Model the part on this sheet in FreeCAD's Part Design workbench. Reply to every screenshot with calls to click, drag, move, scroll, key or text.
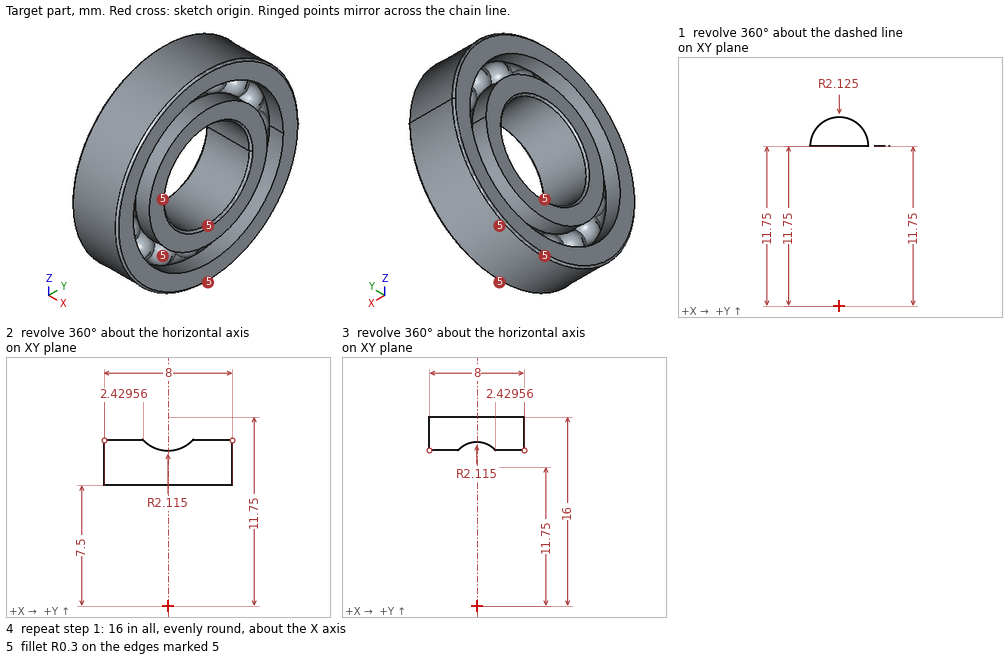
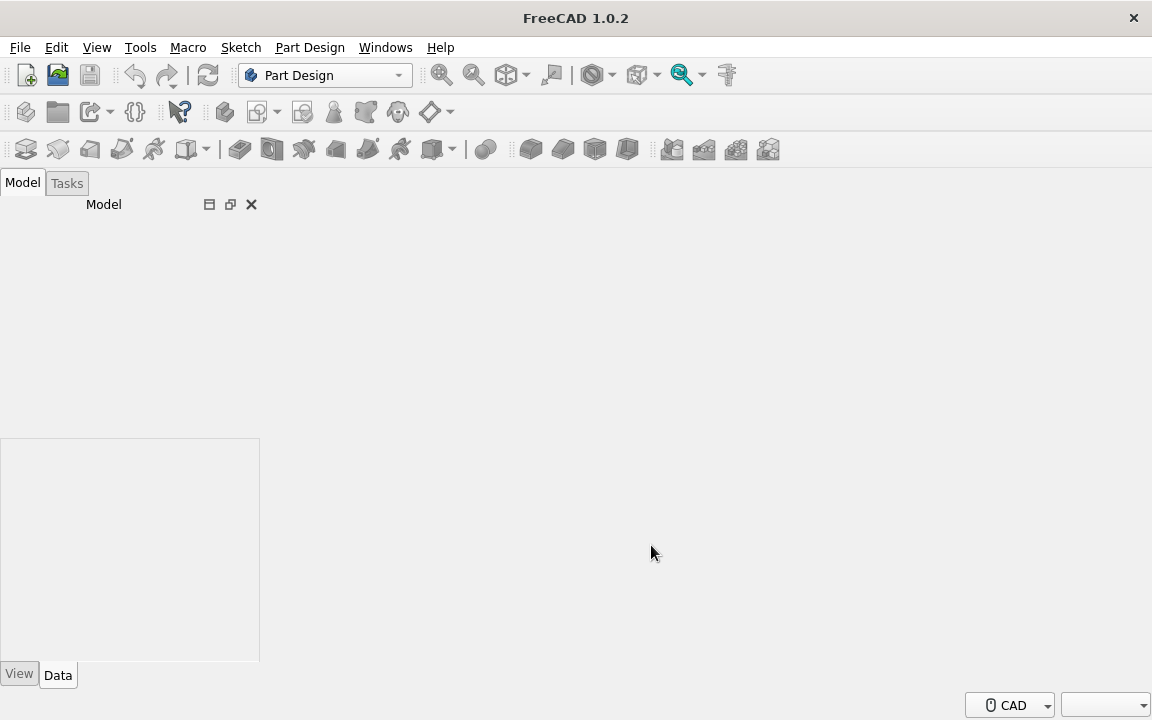
click(26, 76)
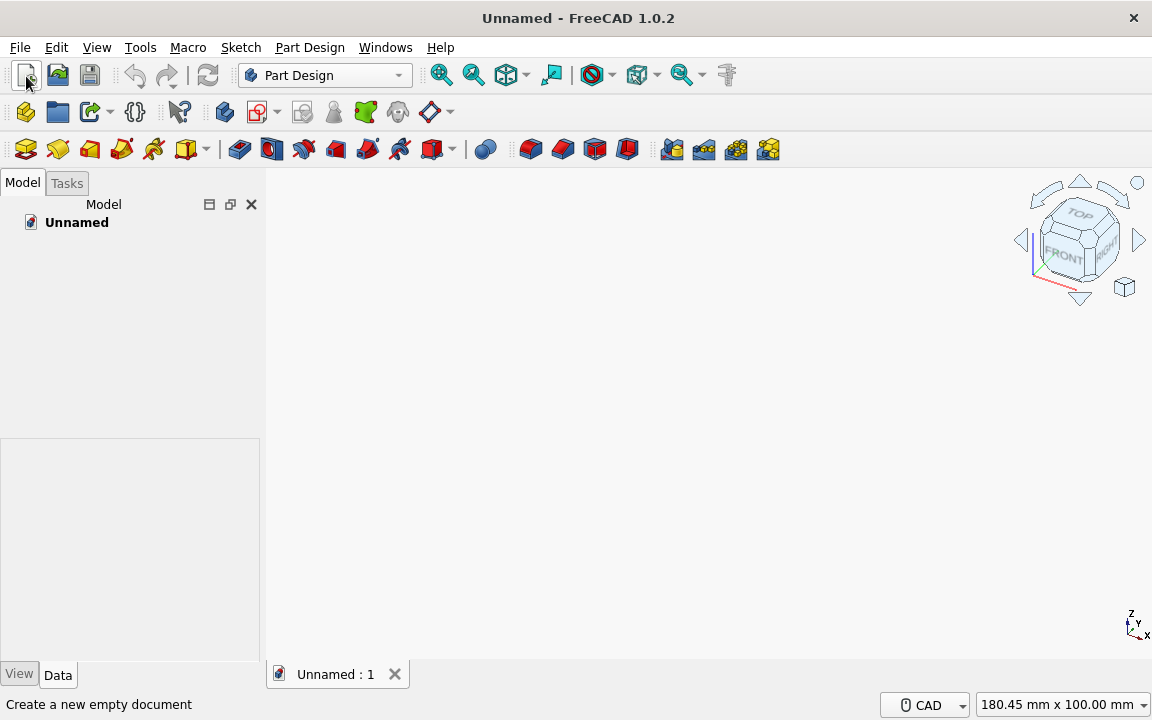
click(258, 112)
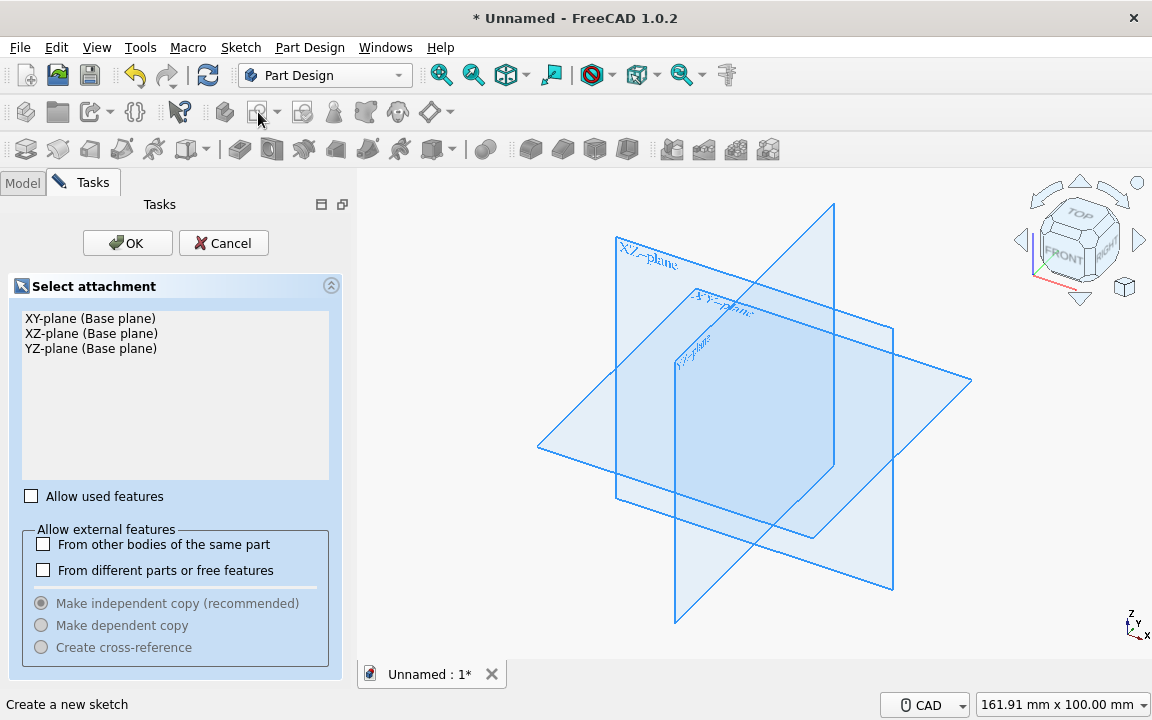
click(82, 318)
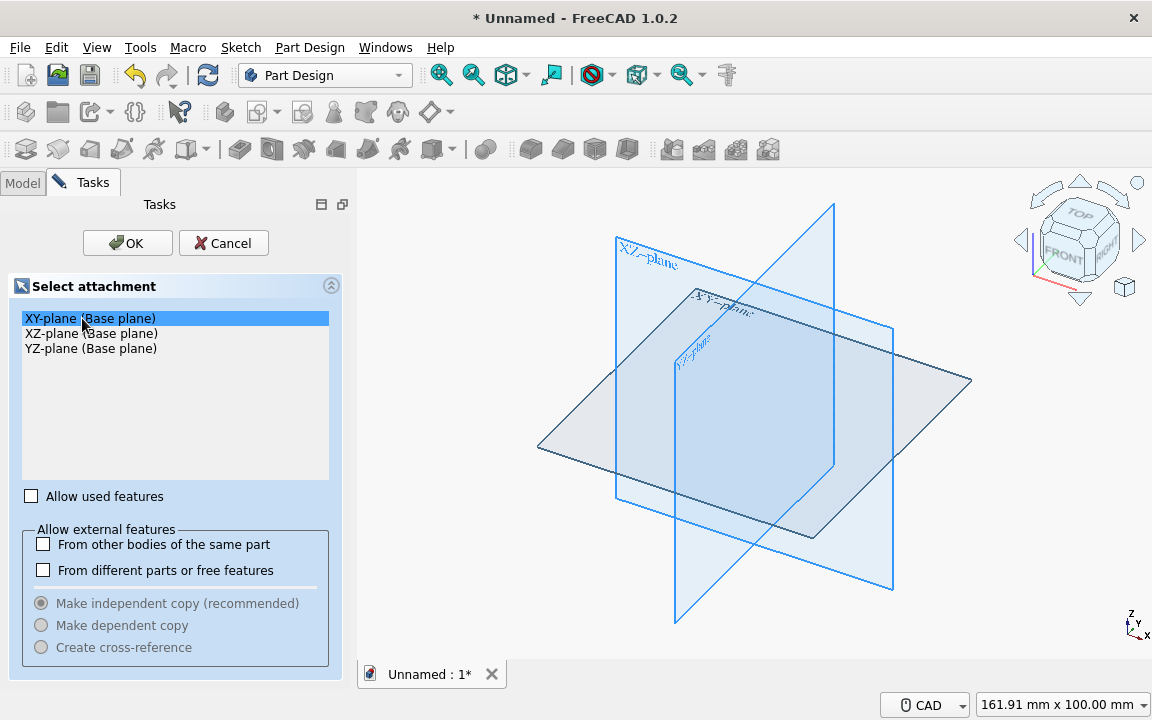
click(128, 243)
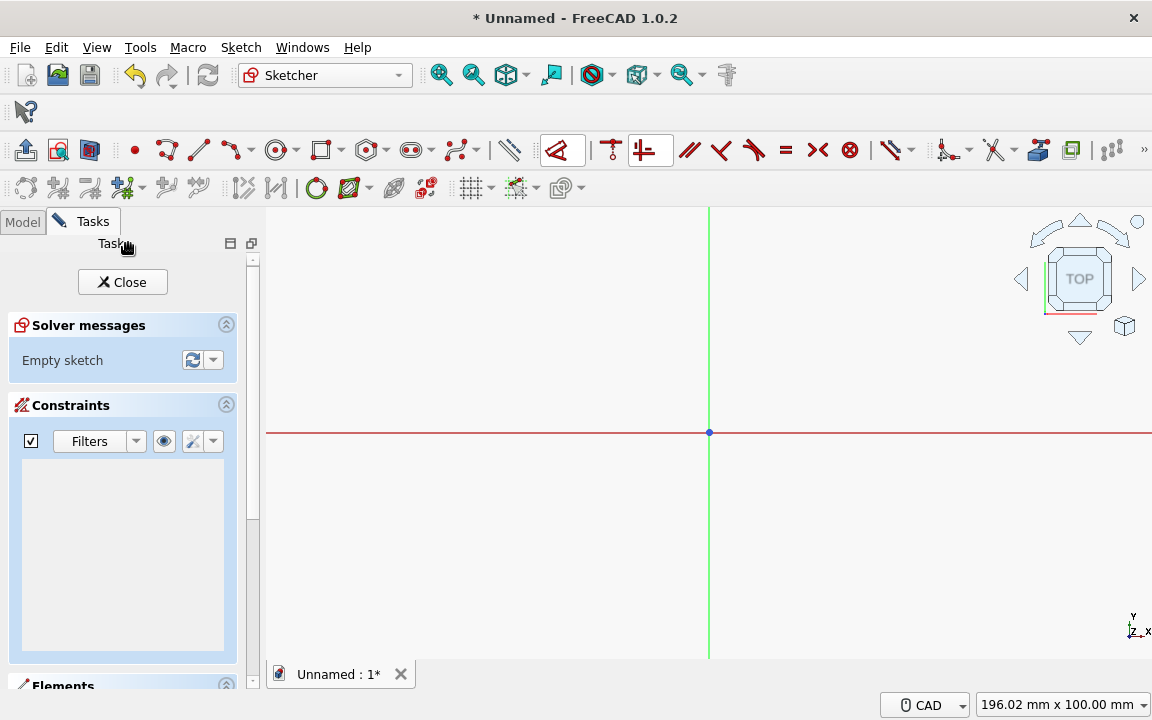
scroll(737, 391, up, 7)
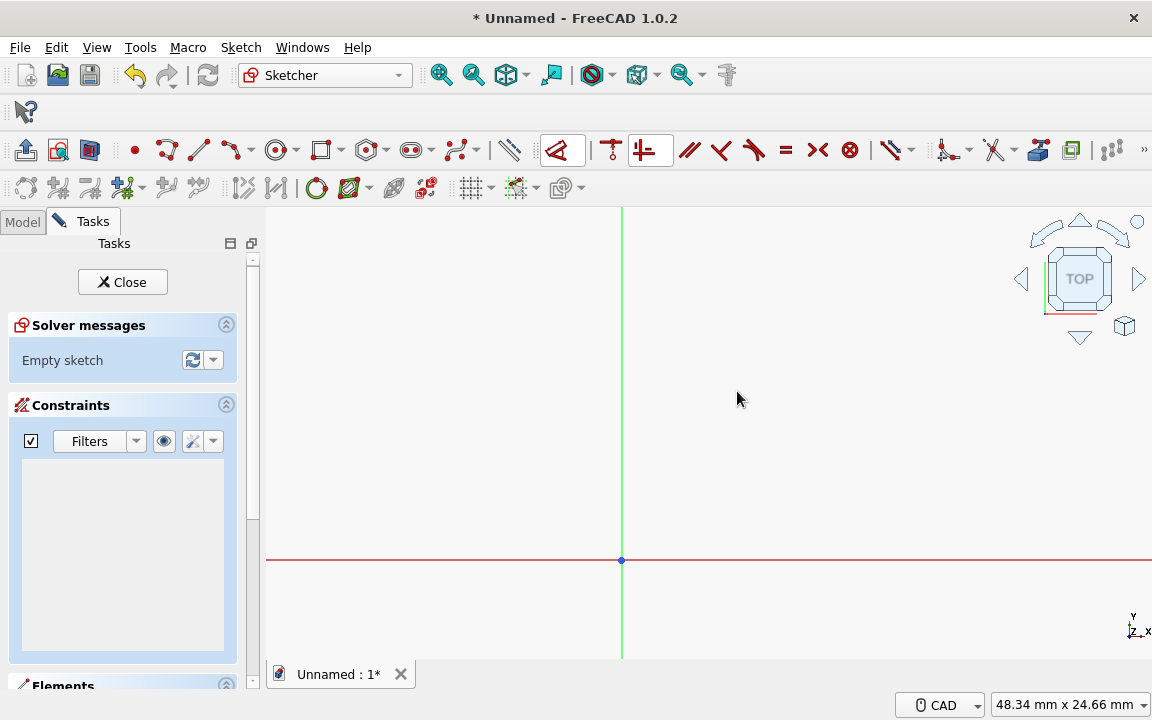
click(200, 150)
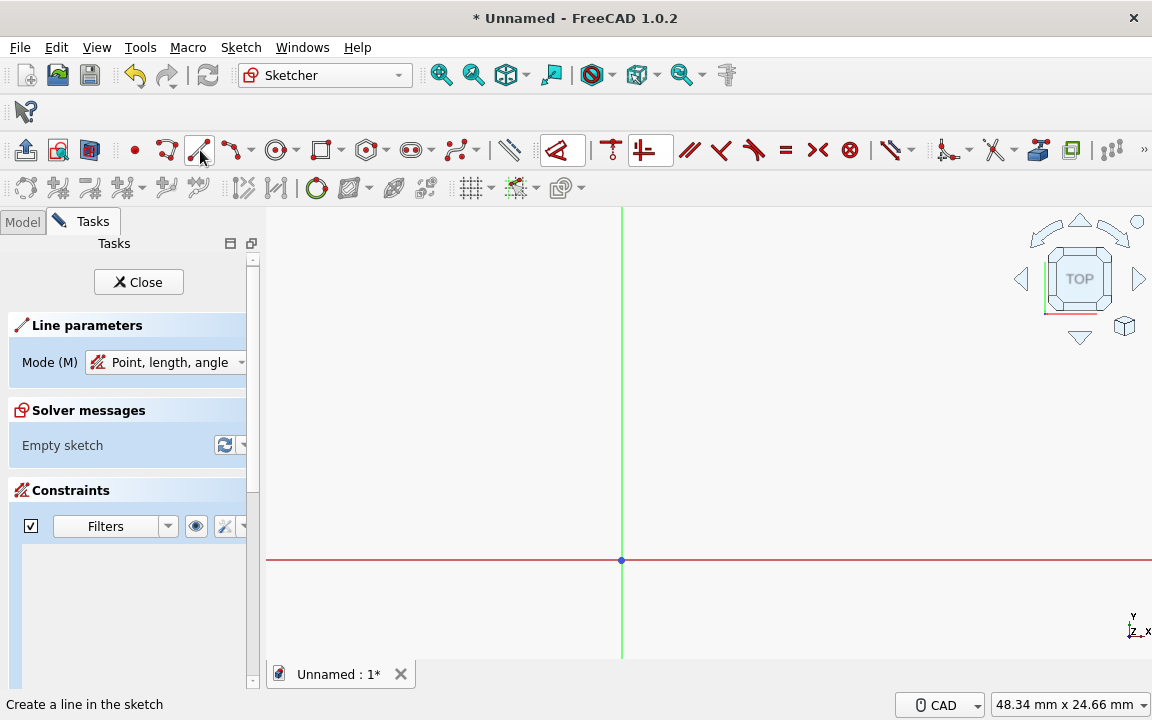
click(583, 345)
click(661, 345)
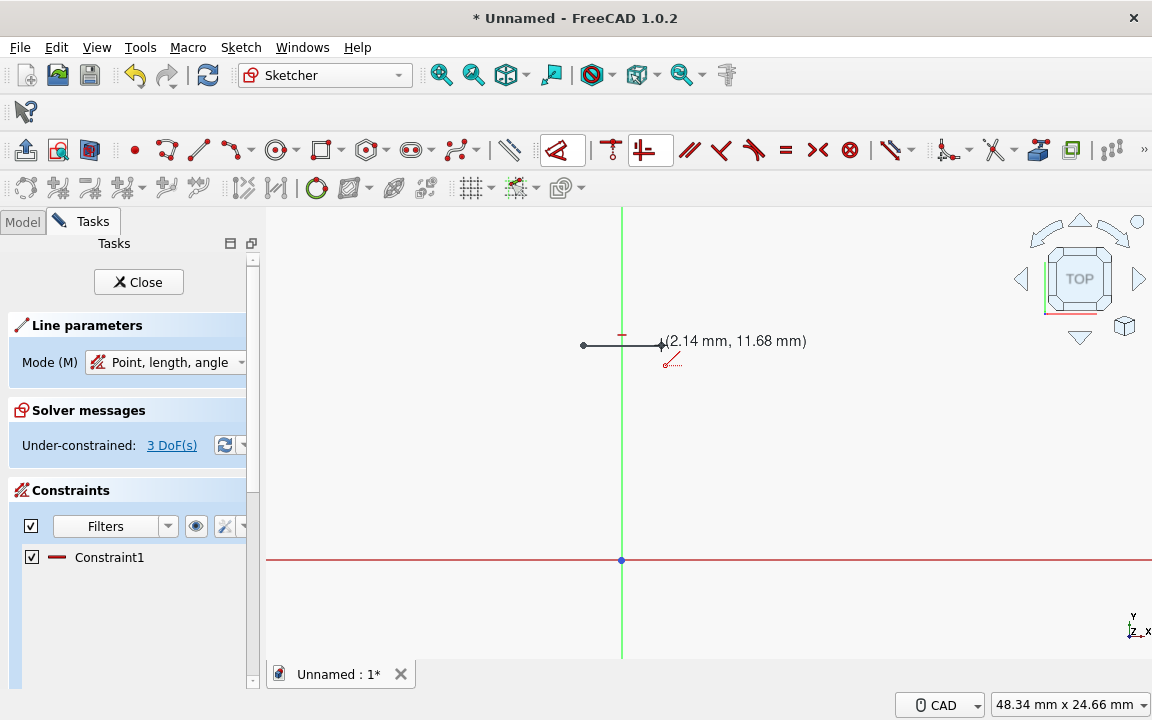
click(232, 150)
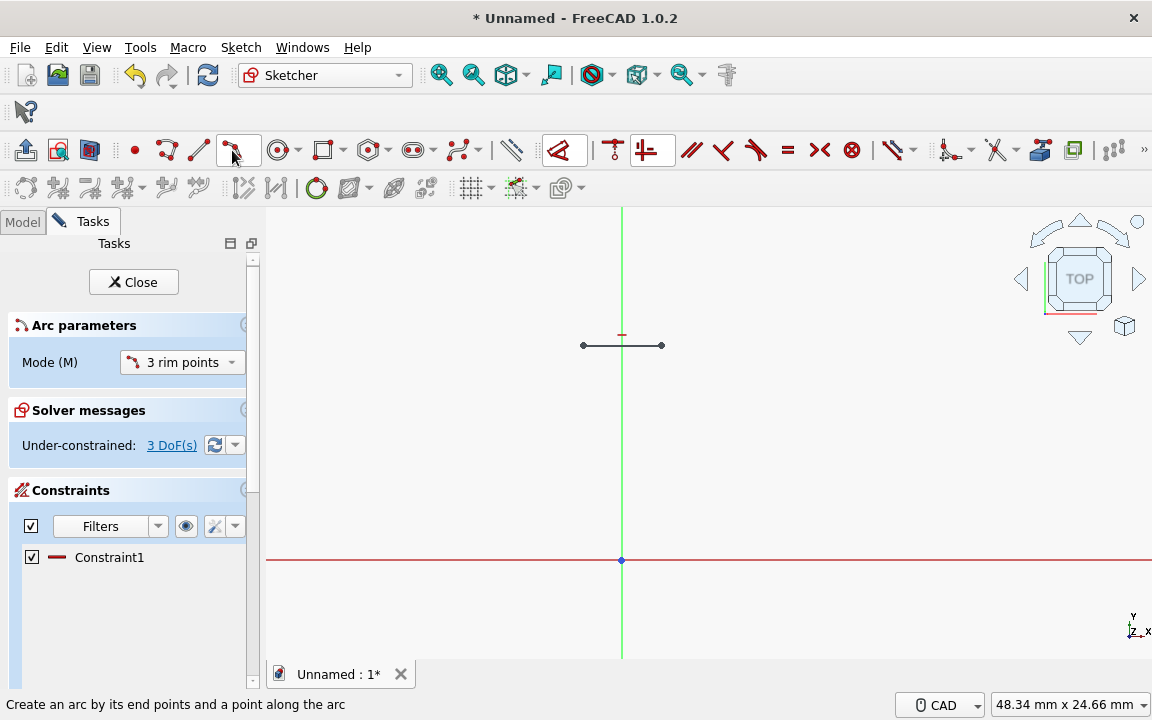
click(661, 346)
click(583, 346)
click(645, 313)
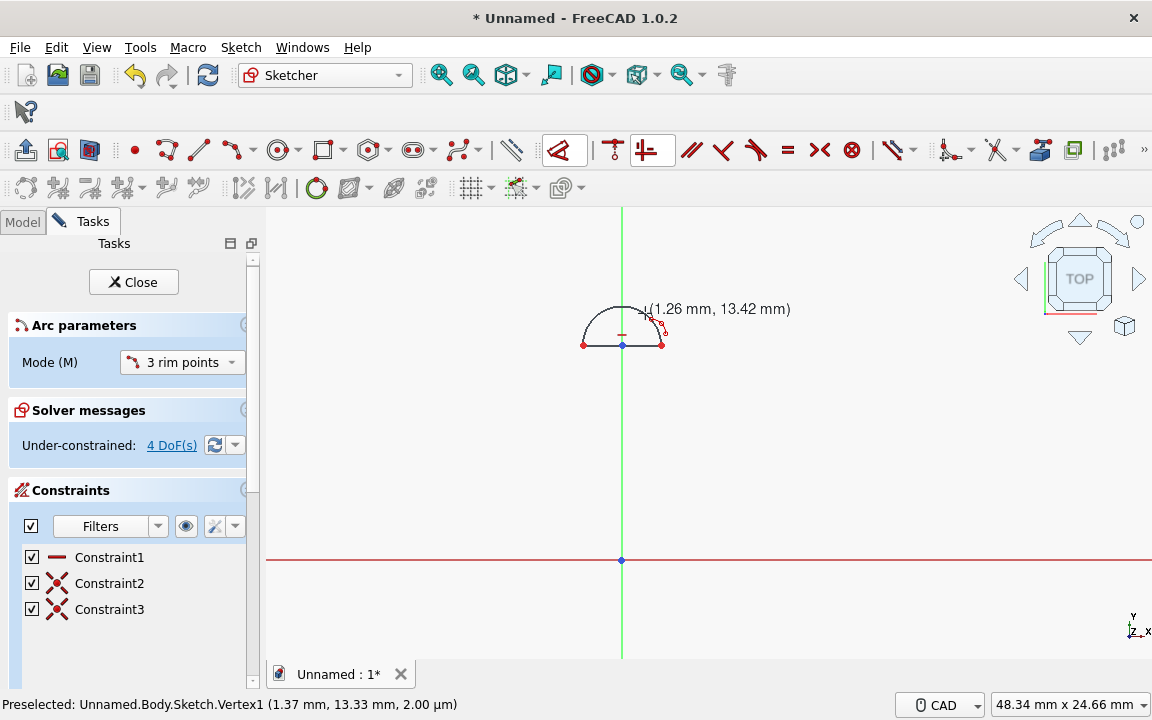
click(200, 150)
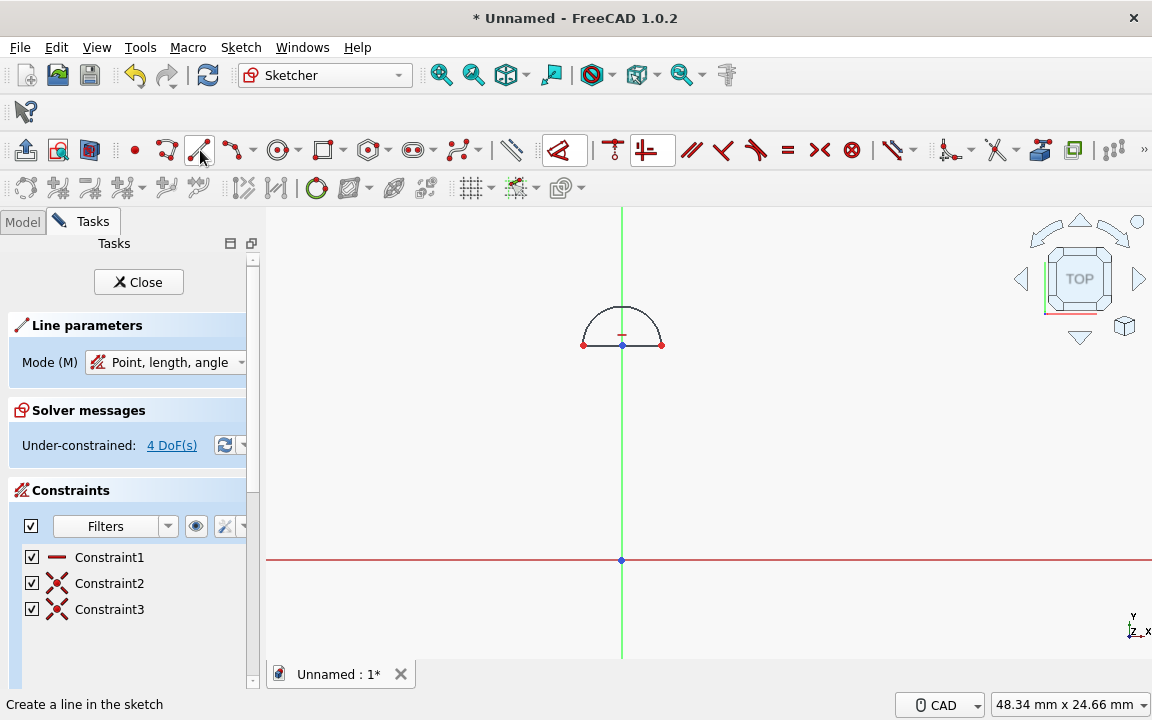
scroll(669, 345, up, 4)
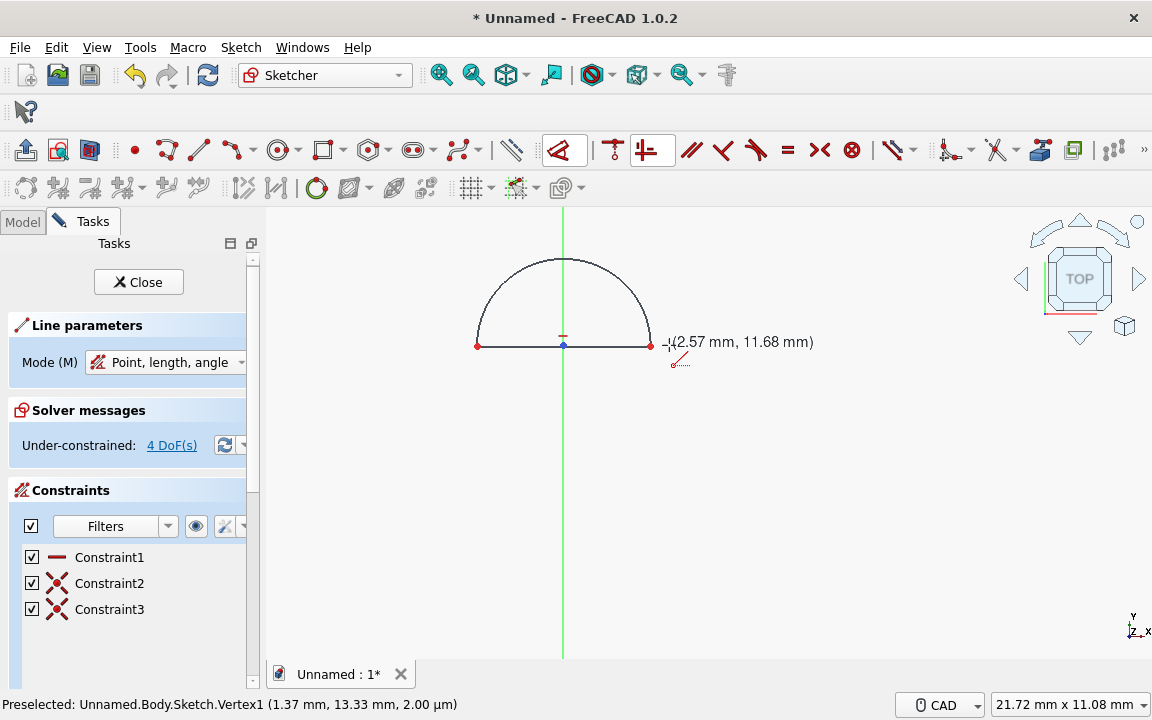
click(667, 344)
click(719, 344)
key(Escape)